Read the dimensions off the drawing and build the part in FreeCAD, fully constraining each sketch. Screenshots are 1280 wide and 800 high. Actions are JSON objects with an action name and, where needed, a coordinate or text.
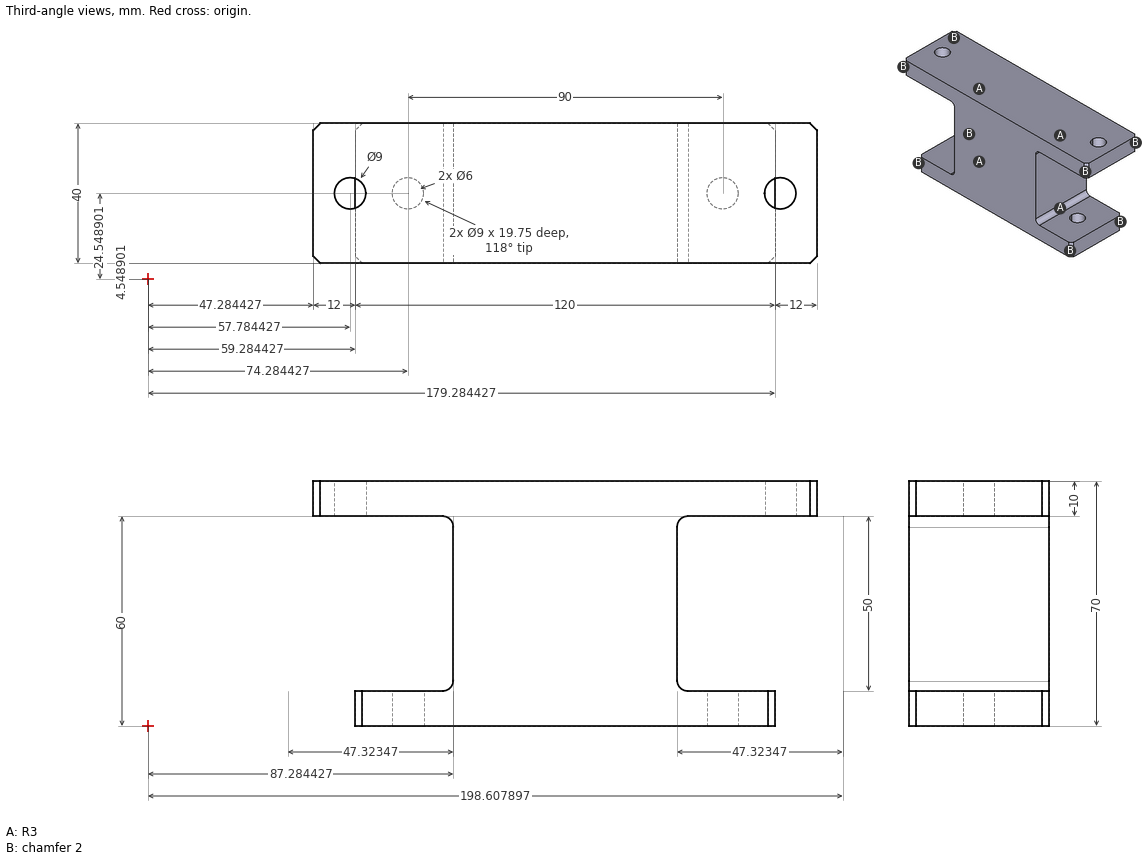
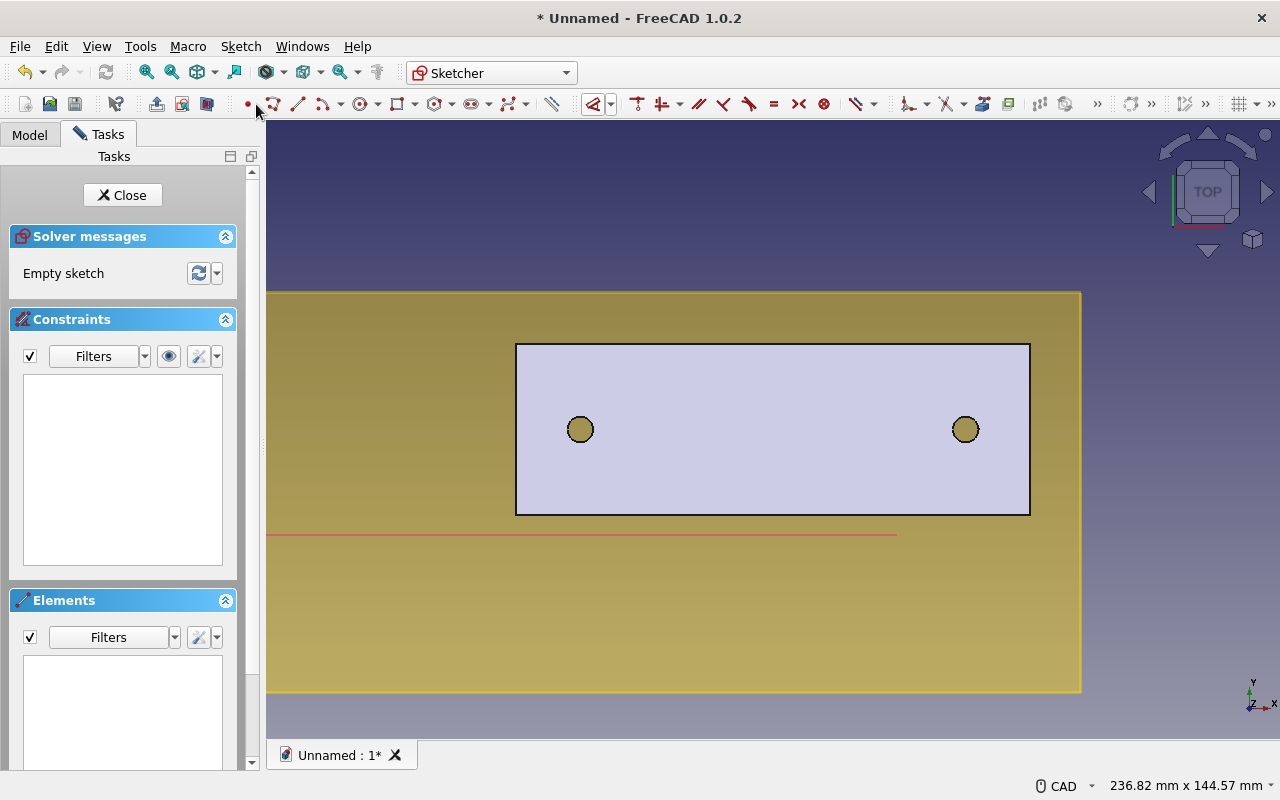
{"action": "key", "text": "q s"}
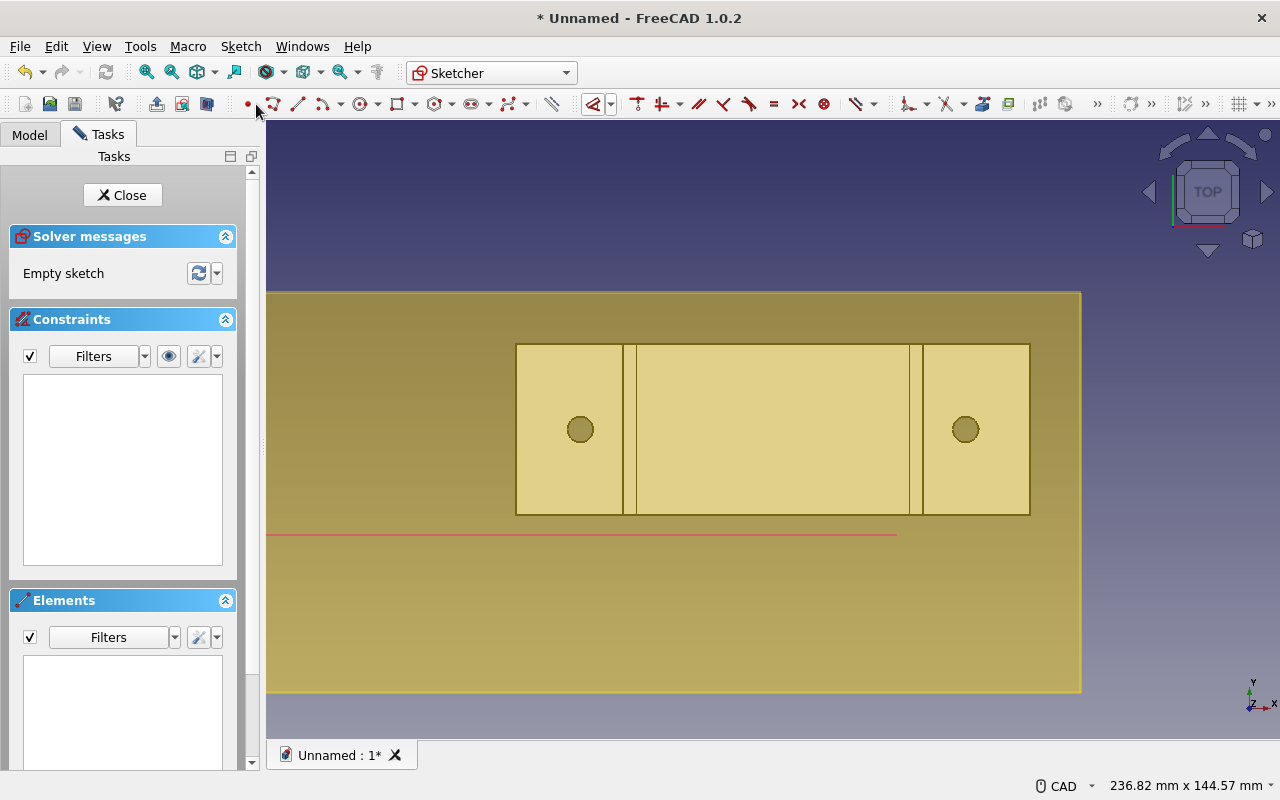
{"action": "scroll", "coordinate": [1115, 430], "scroll_direction": "up", "scroll_amount": 4}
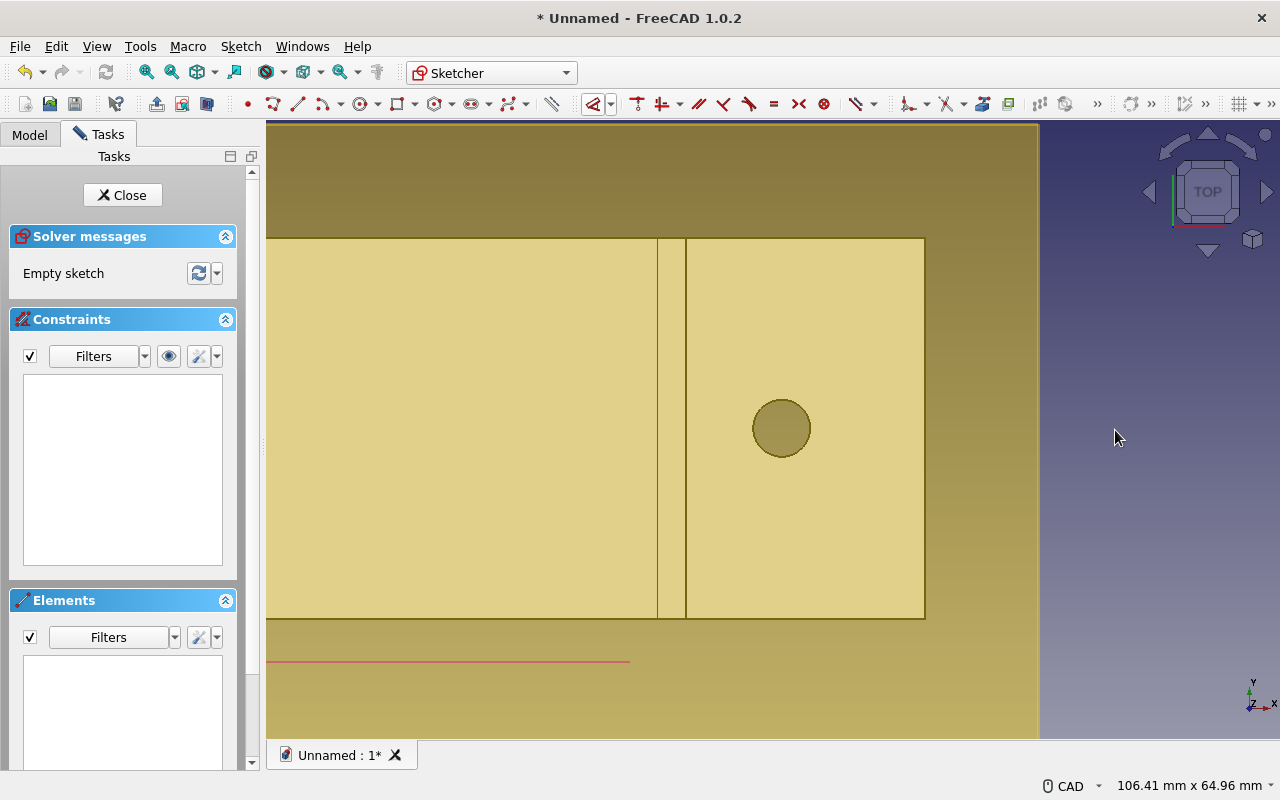
{"action": "key", "text": "g r"}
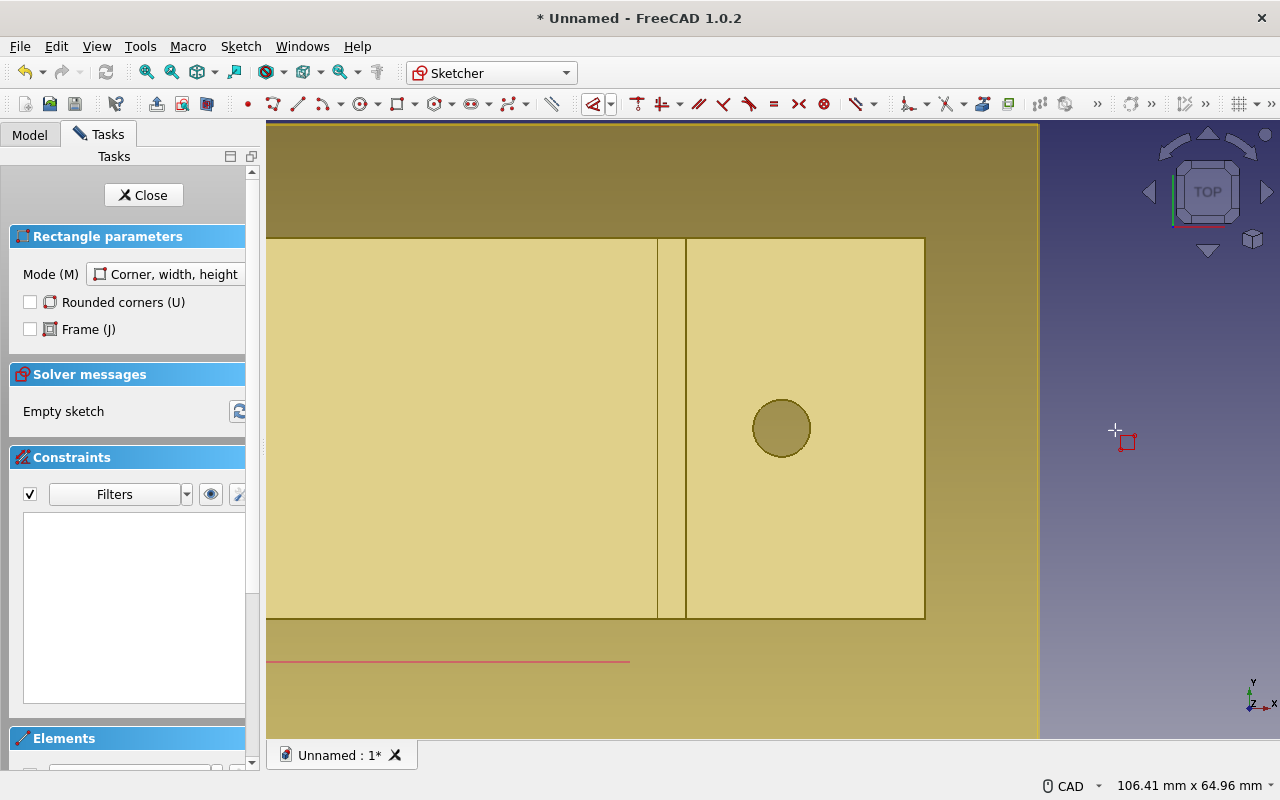
{"action": "left_click", "coordinate": [925, 238]}
{"action": "left_click", "coordinate": [1039, 619]}
{"action": "key", "text": "Escape"}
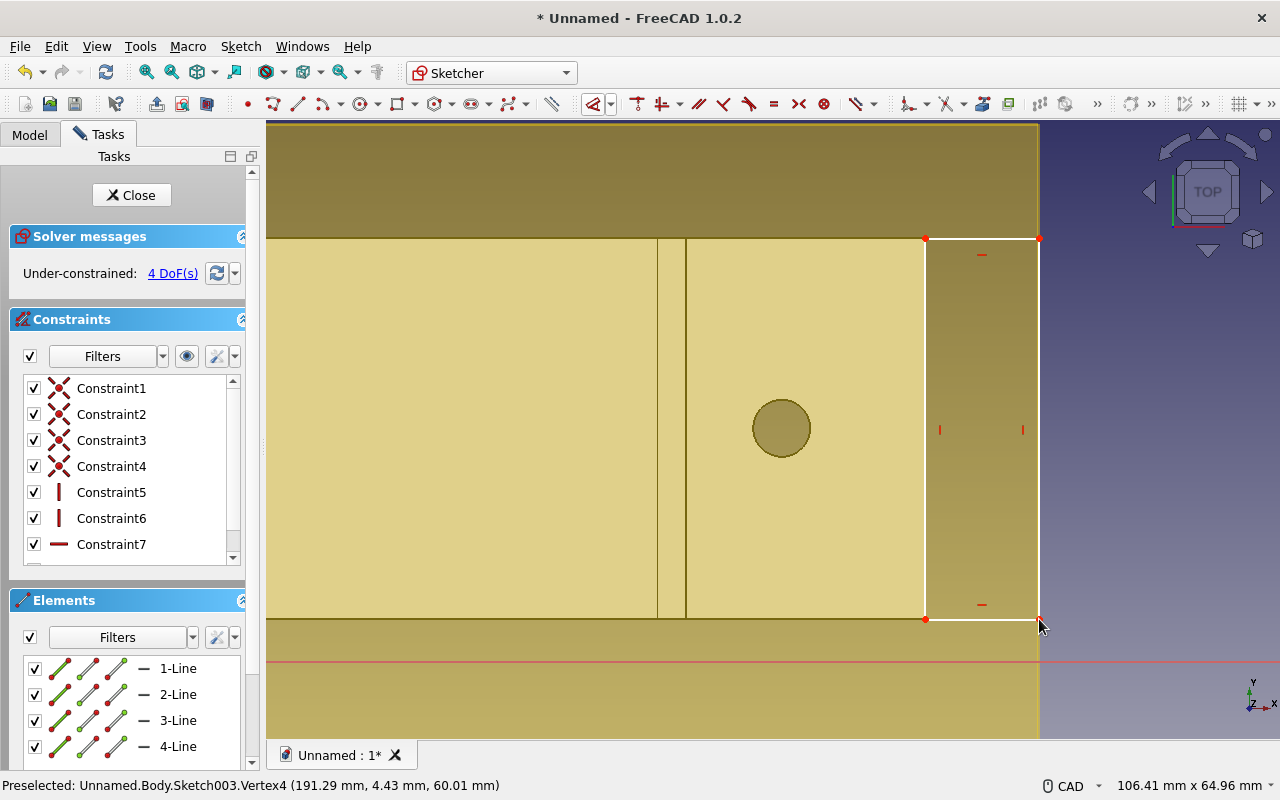
{"action": "left_click", "coordinate": [925, 353]}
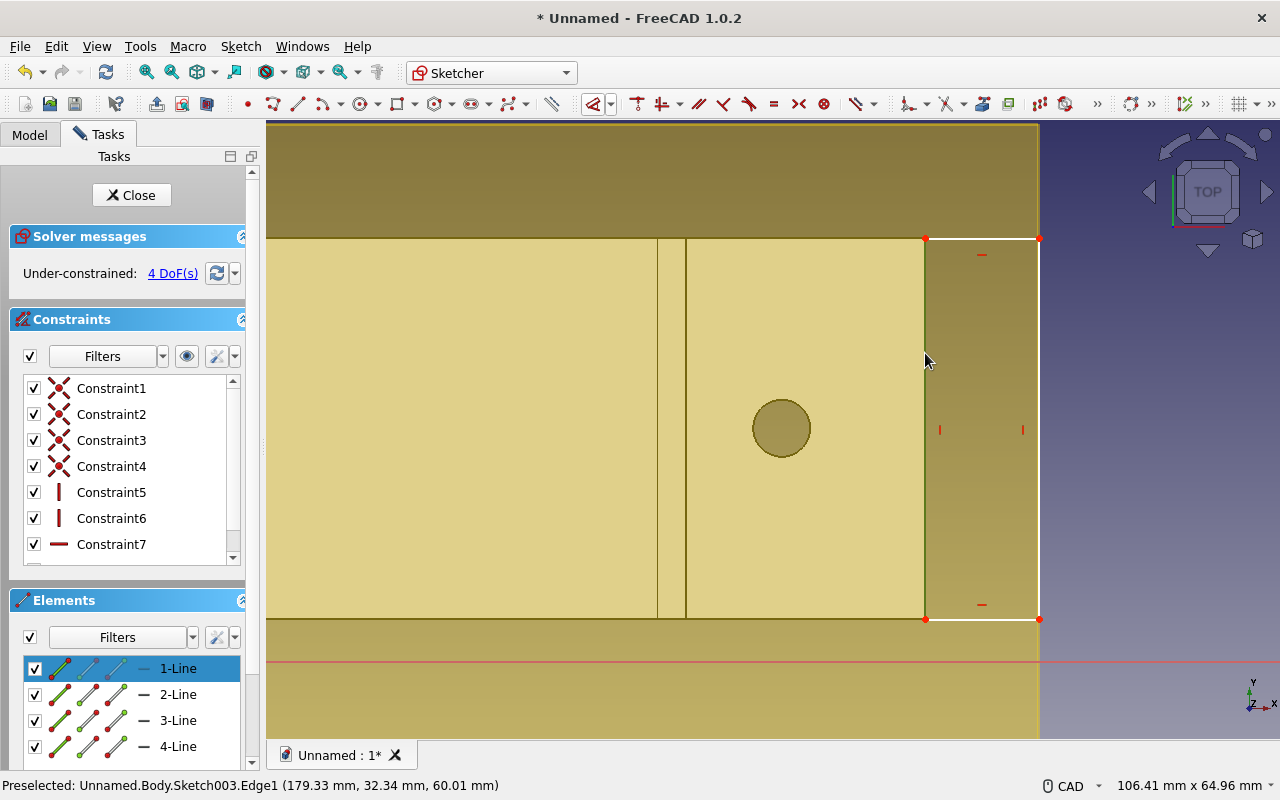
{"action": "key", "text": "i"}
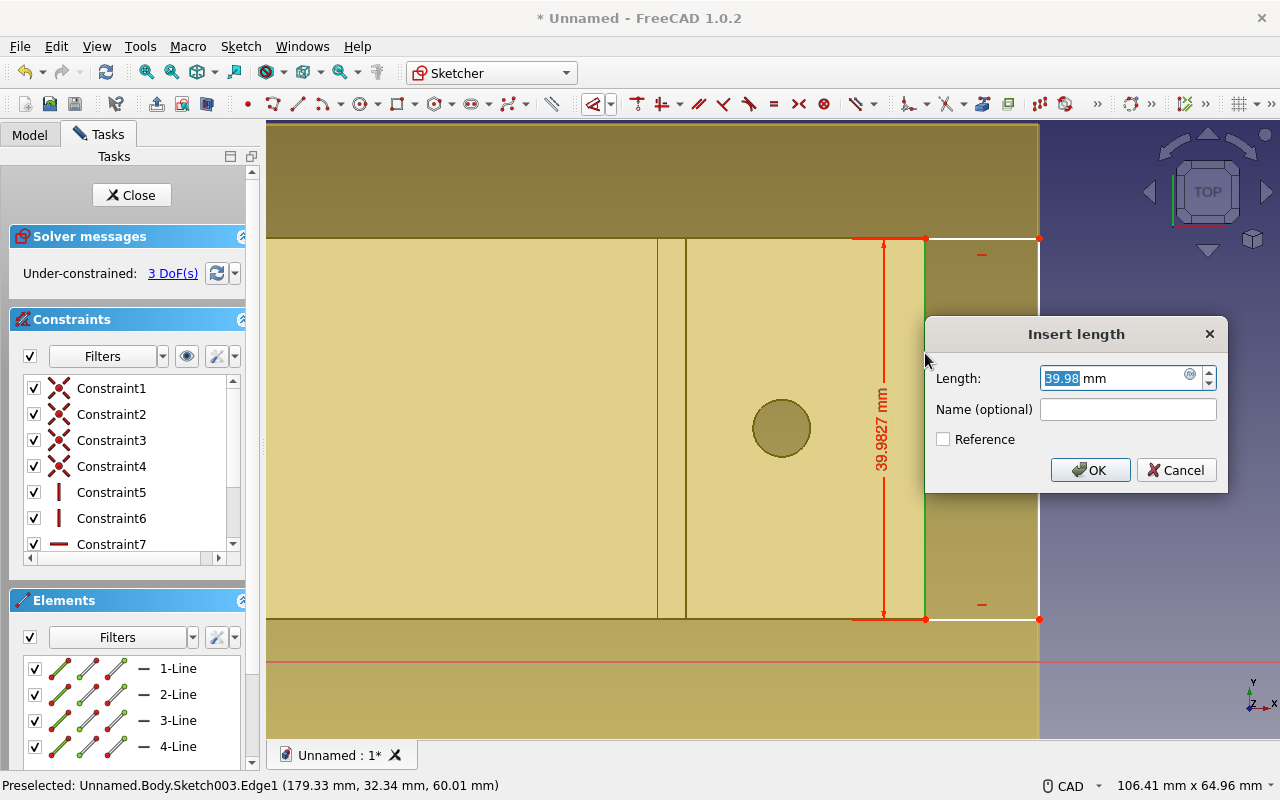
{"action": "type", "text": "40"}
{"action": "key", "text": "Return"}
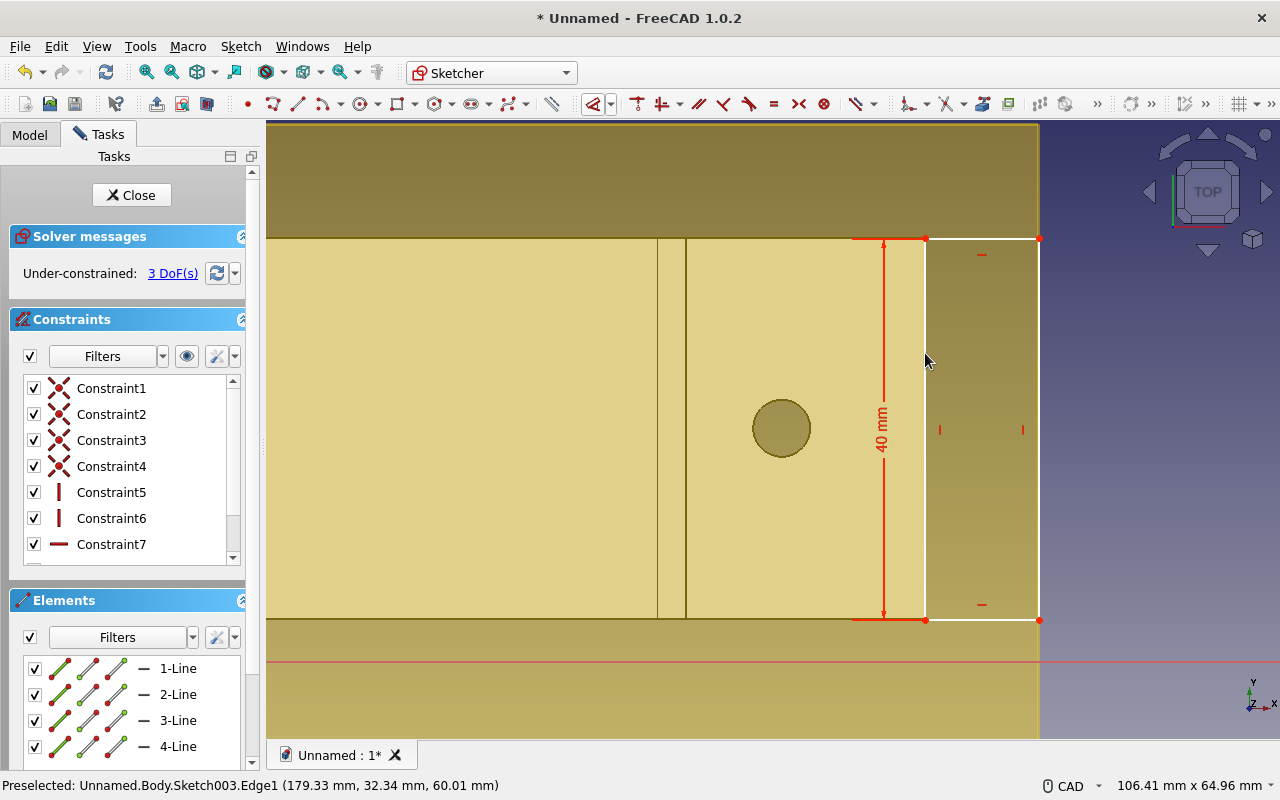
{"action": "left_click", "coordinate": [959, 620]}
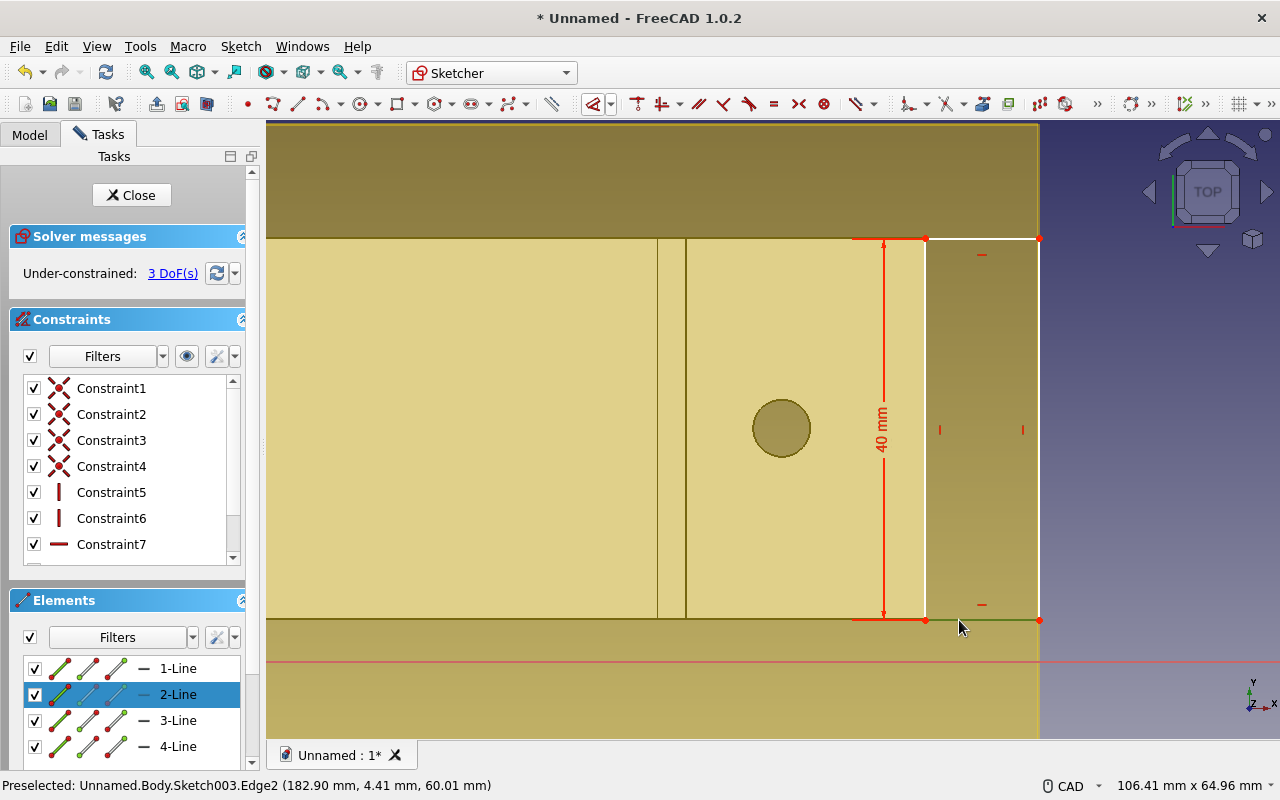
{"action": "left_click", "coordinate": [610, 104]}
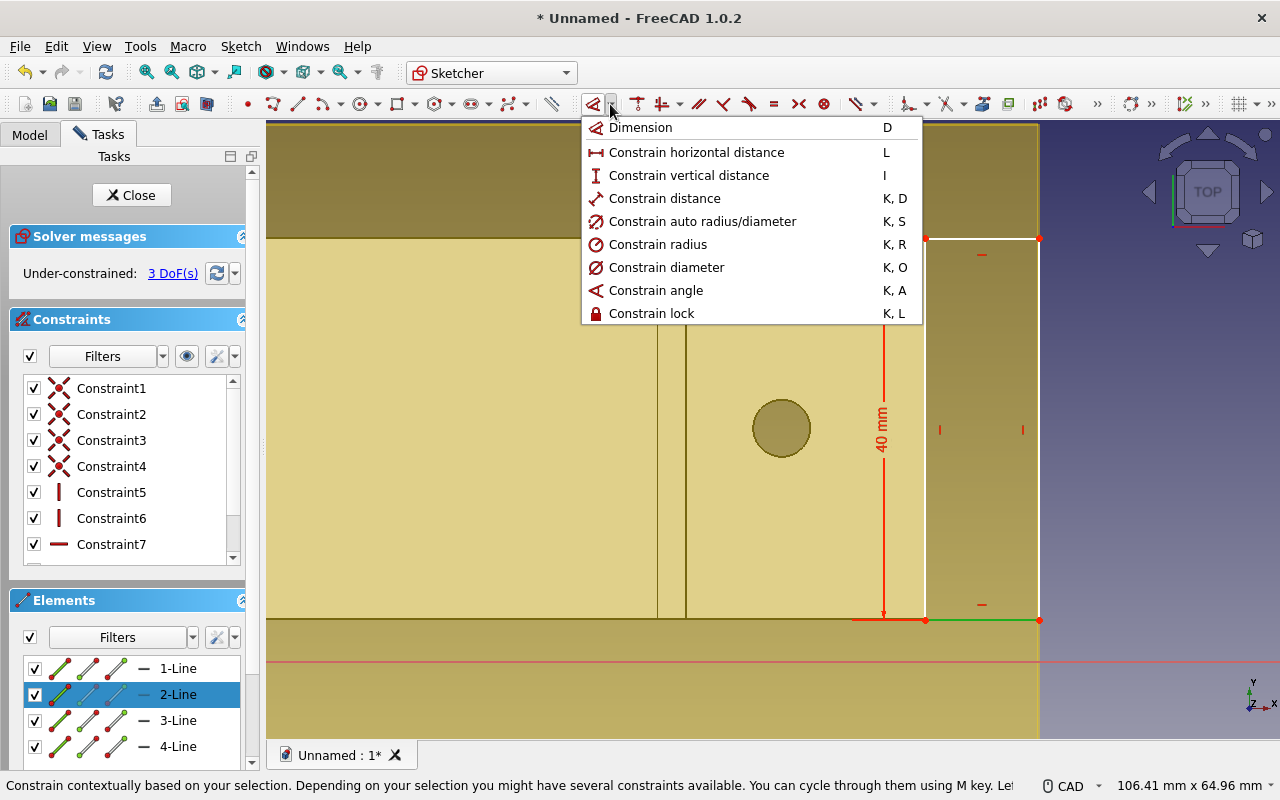
{"action": "left_click", "coordinate": [752, 152]}